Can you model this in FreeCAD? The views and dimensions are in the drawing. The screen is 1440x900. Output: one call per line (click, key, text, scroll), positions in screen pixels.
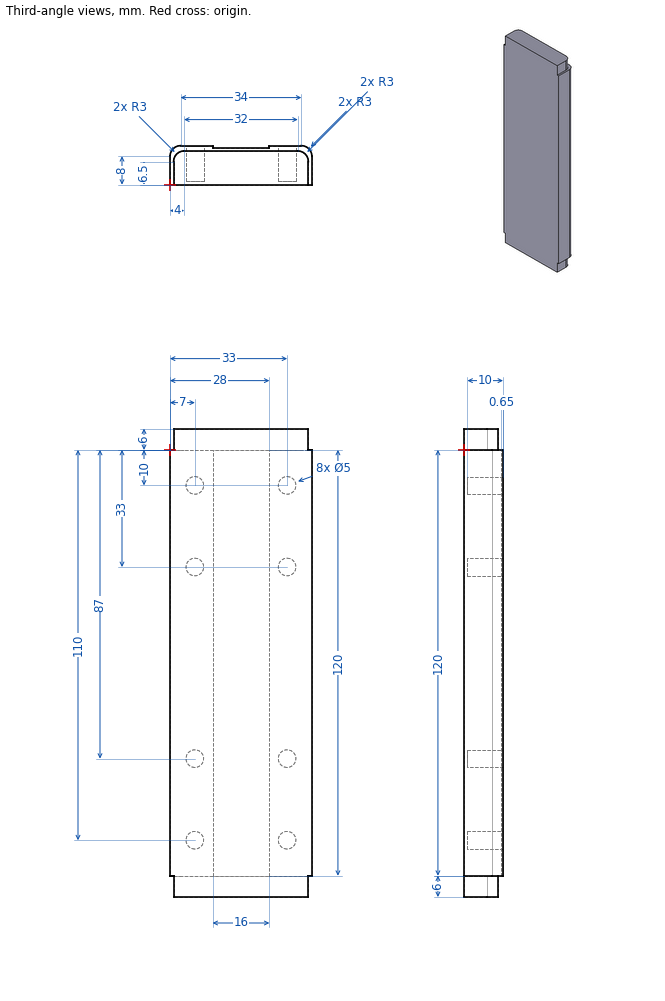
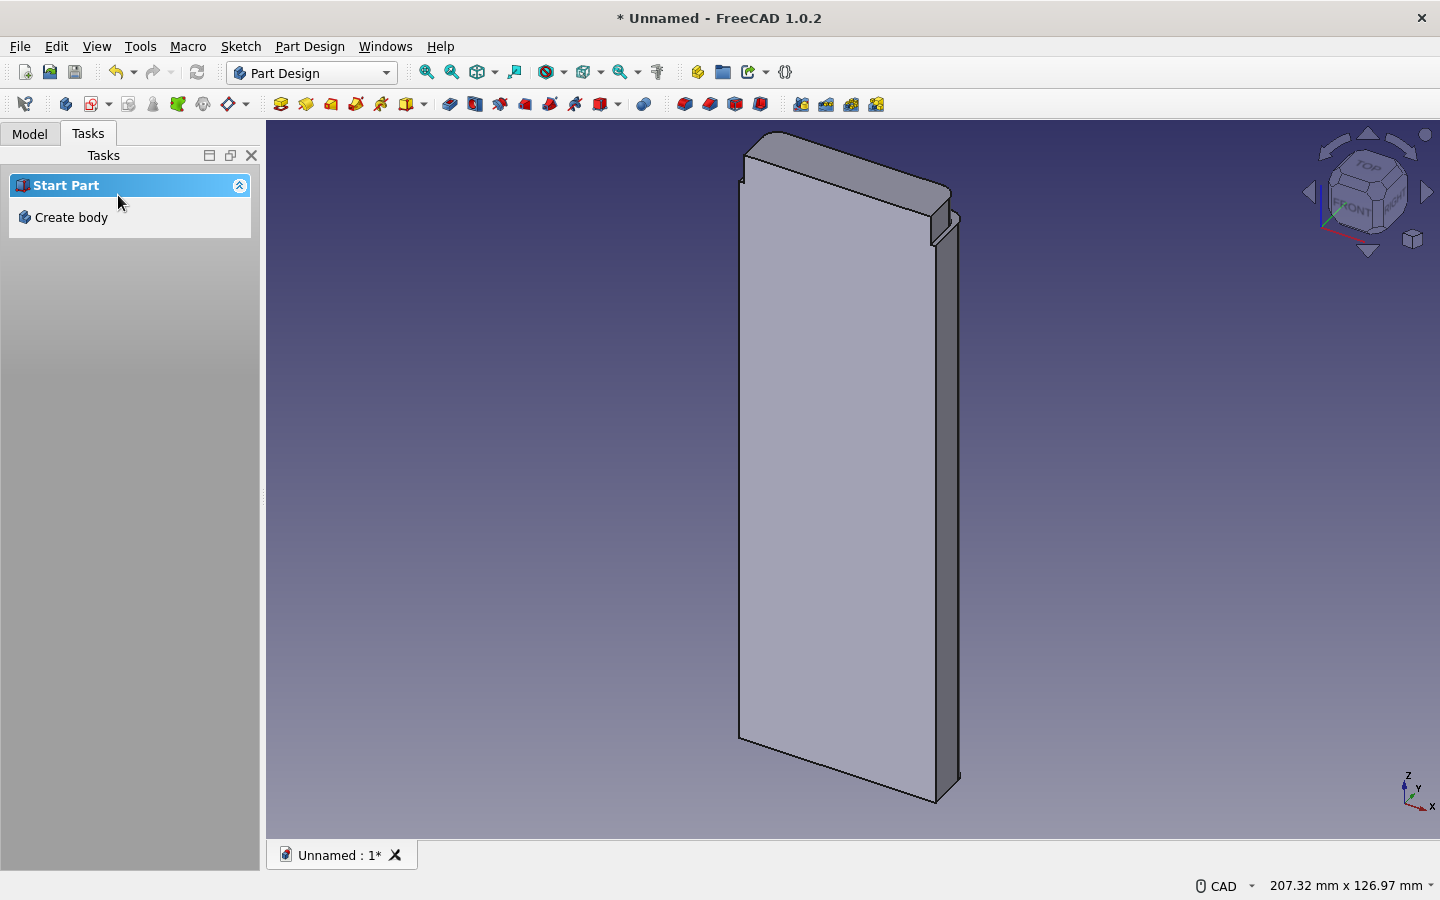
click(30, 134)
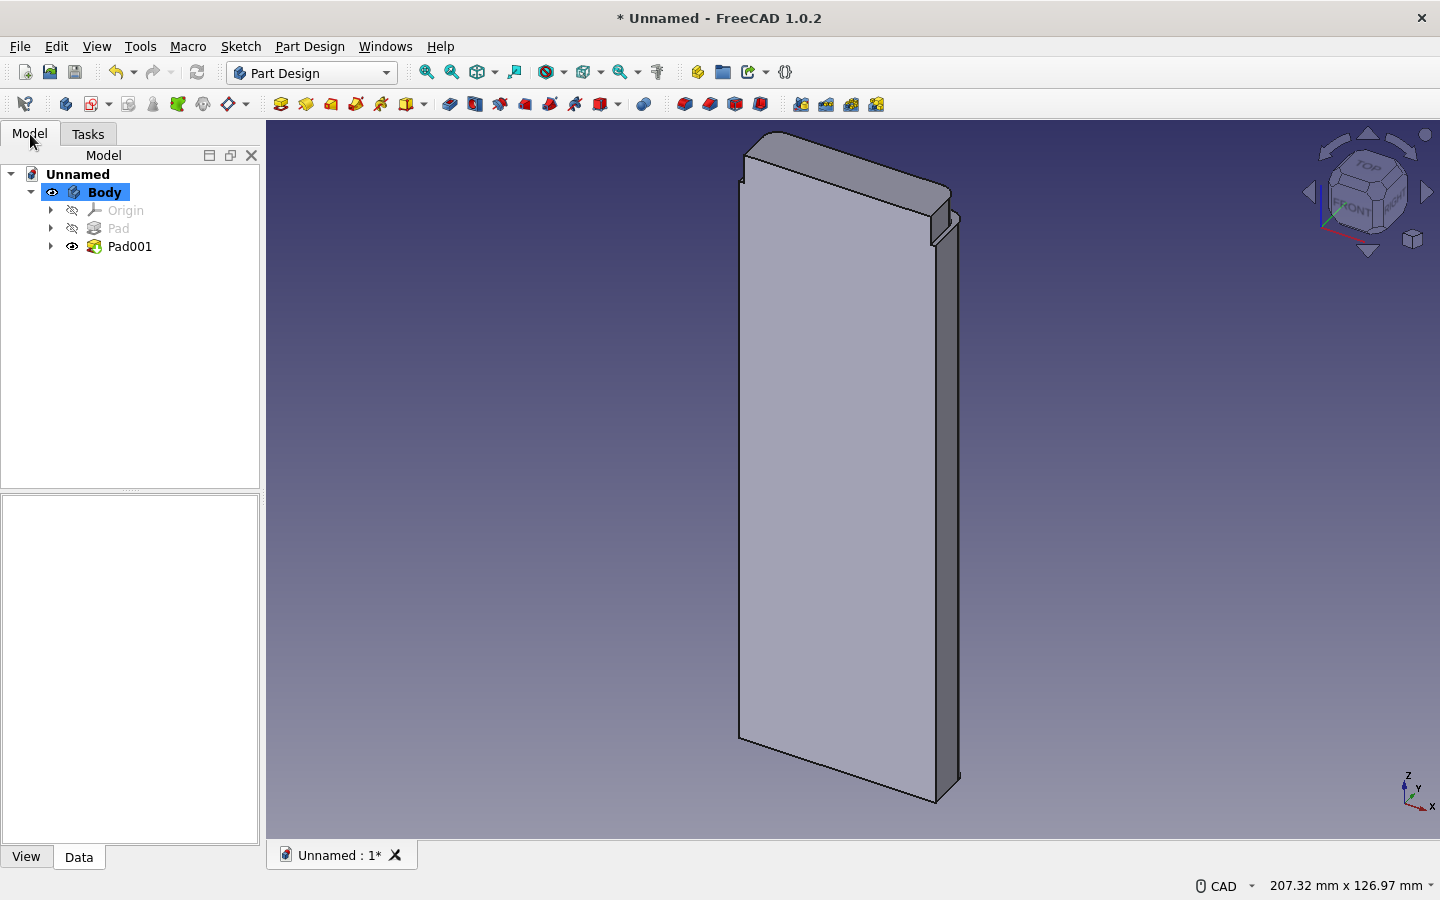
click(51, 210)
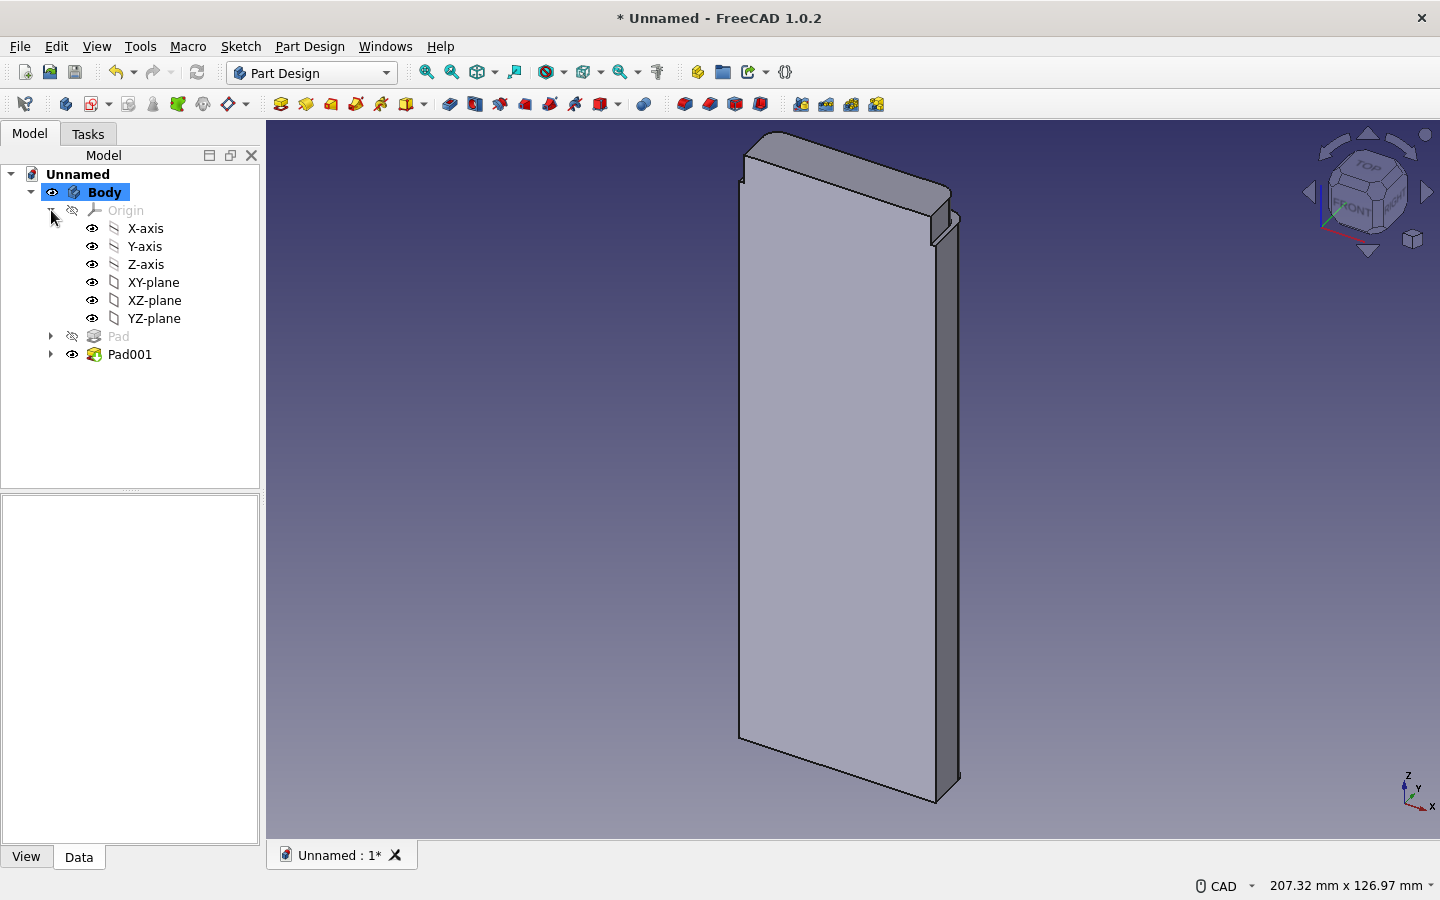
click(137, 282)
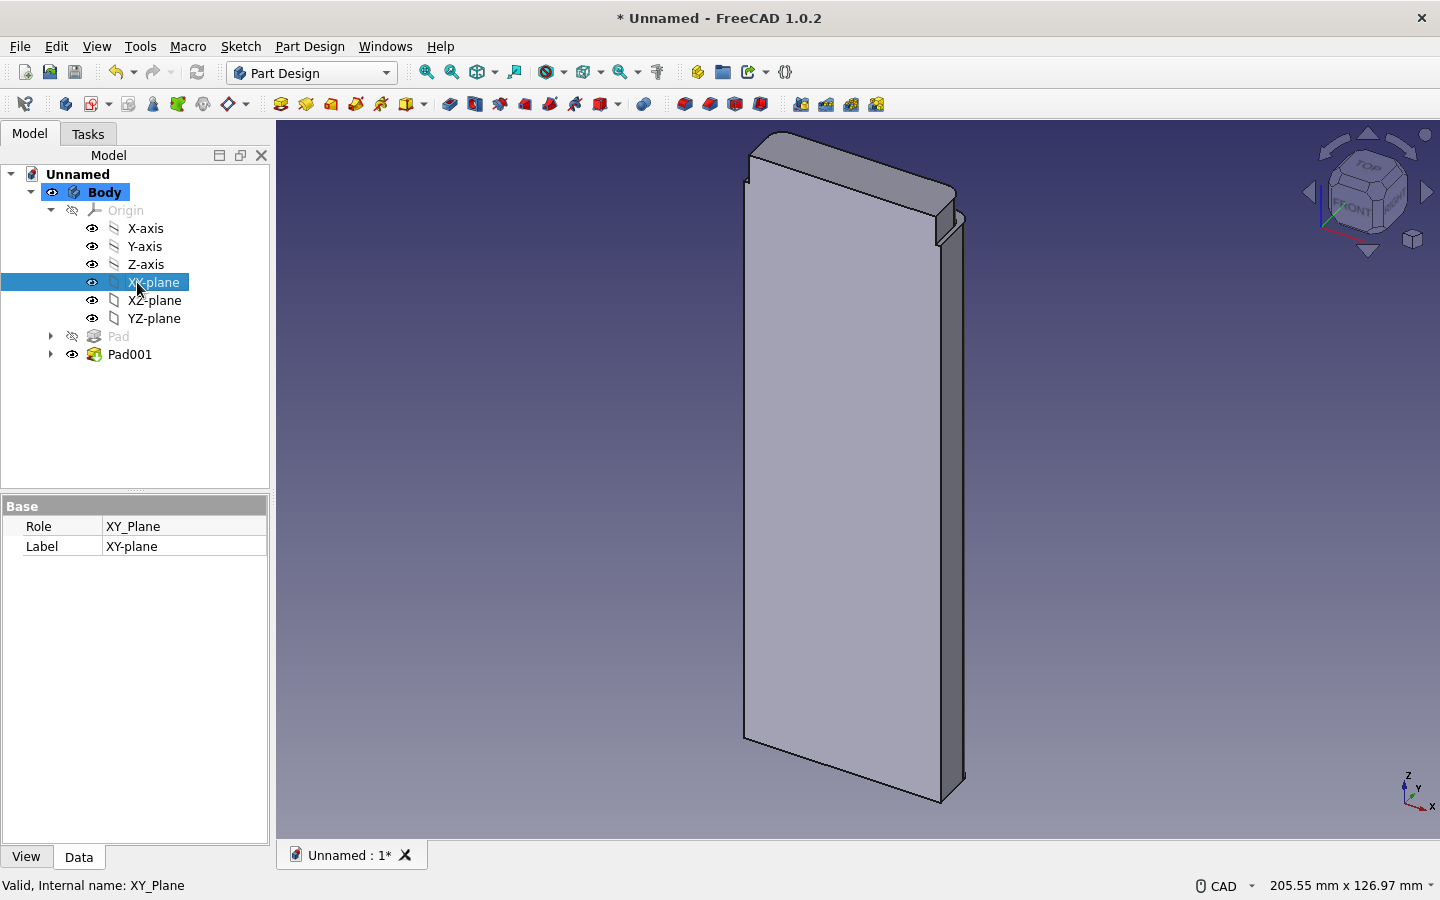
click(228, 104)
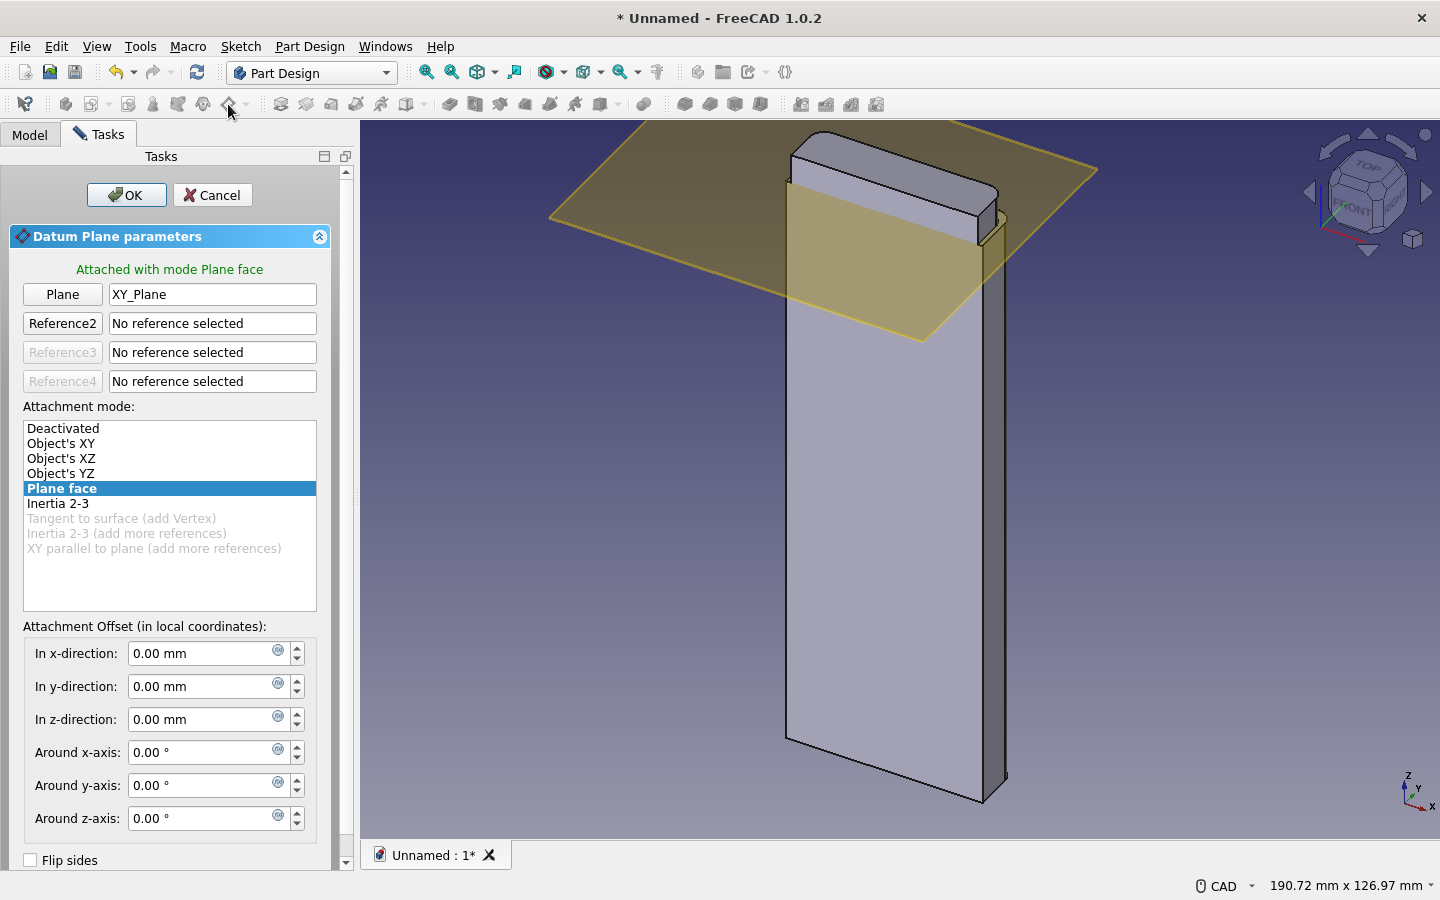
triple_click(210, 720)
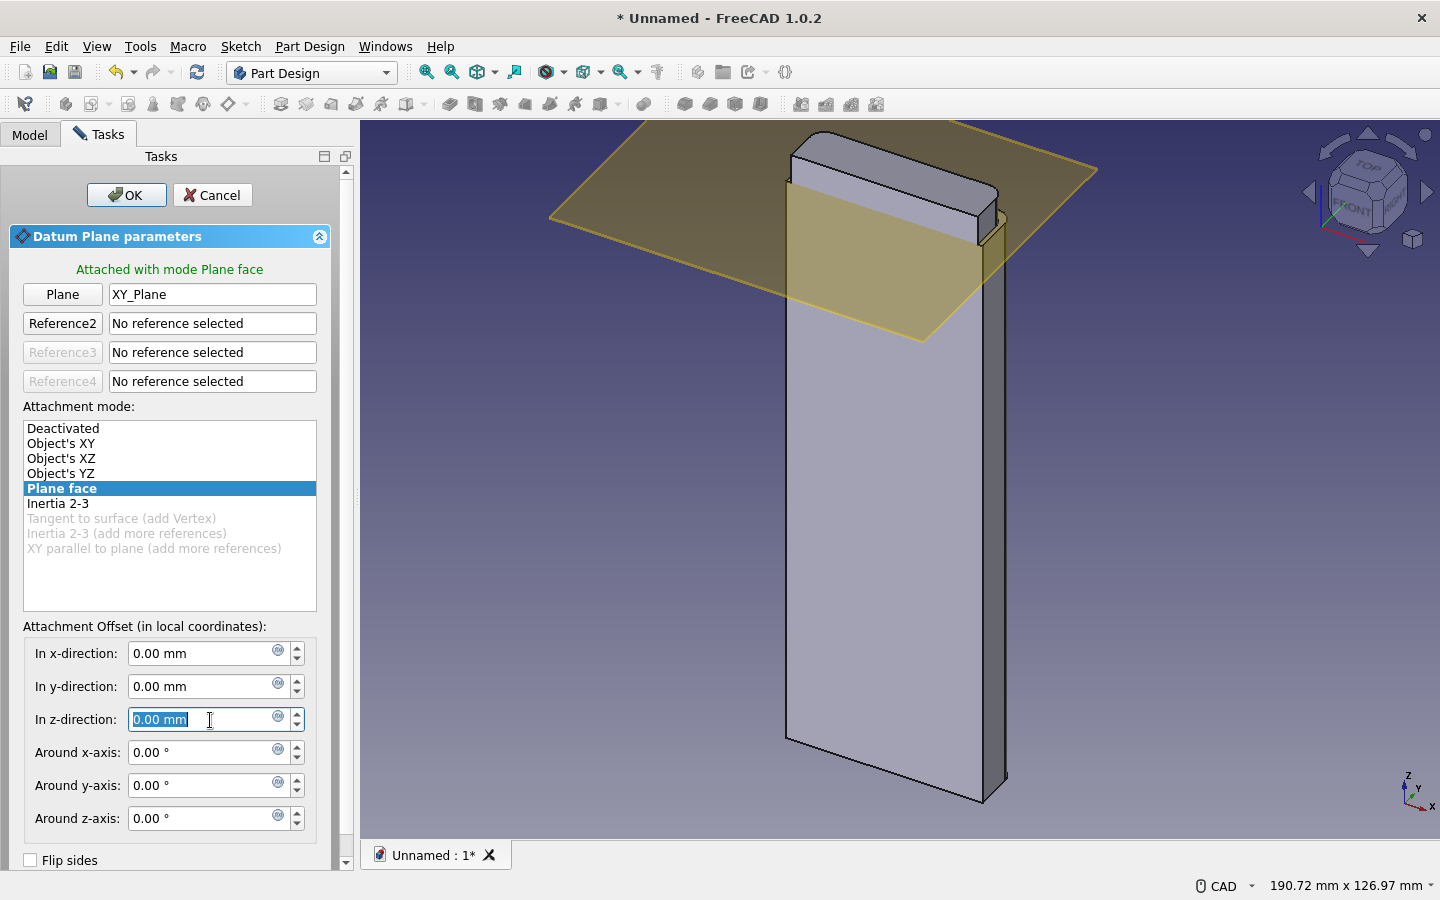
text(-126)
key(Tab)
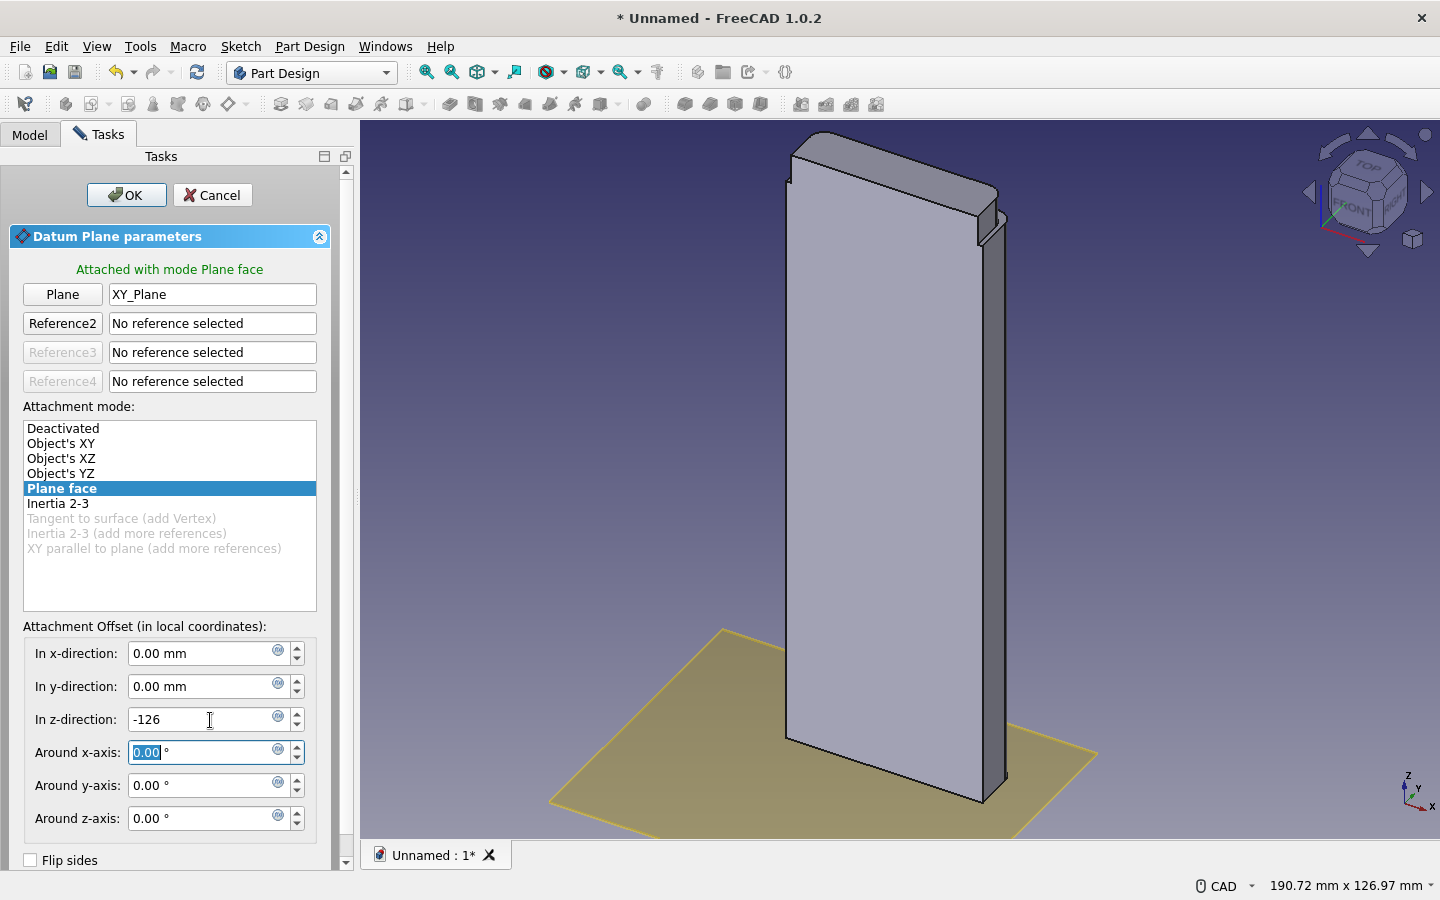
click(127, 195)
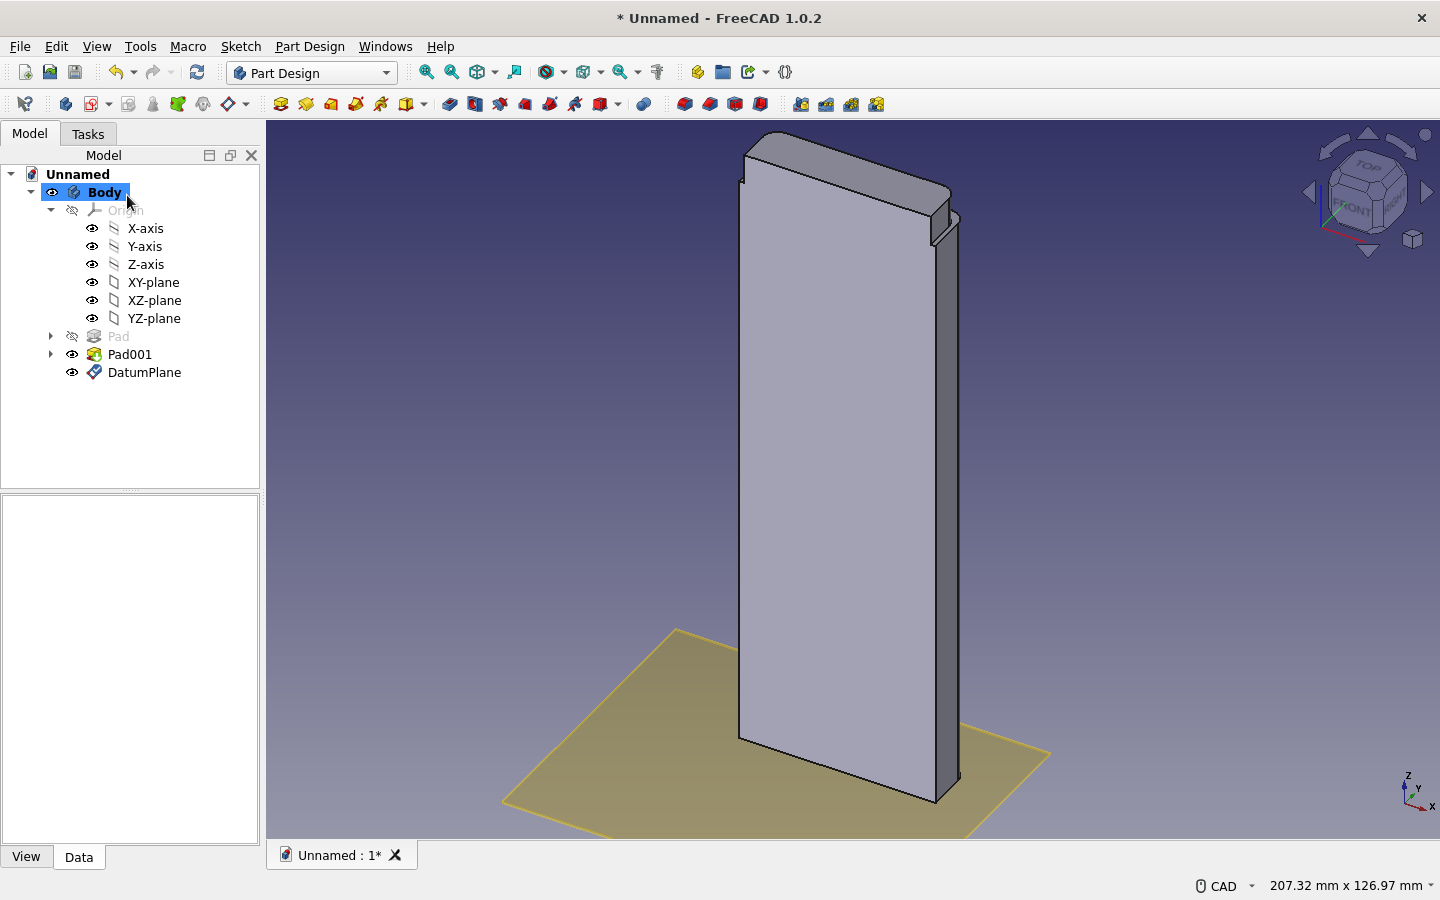
click(117, 372)